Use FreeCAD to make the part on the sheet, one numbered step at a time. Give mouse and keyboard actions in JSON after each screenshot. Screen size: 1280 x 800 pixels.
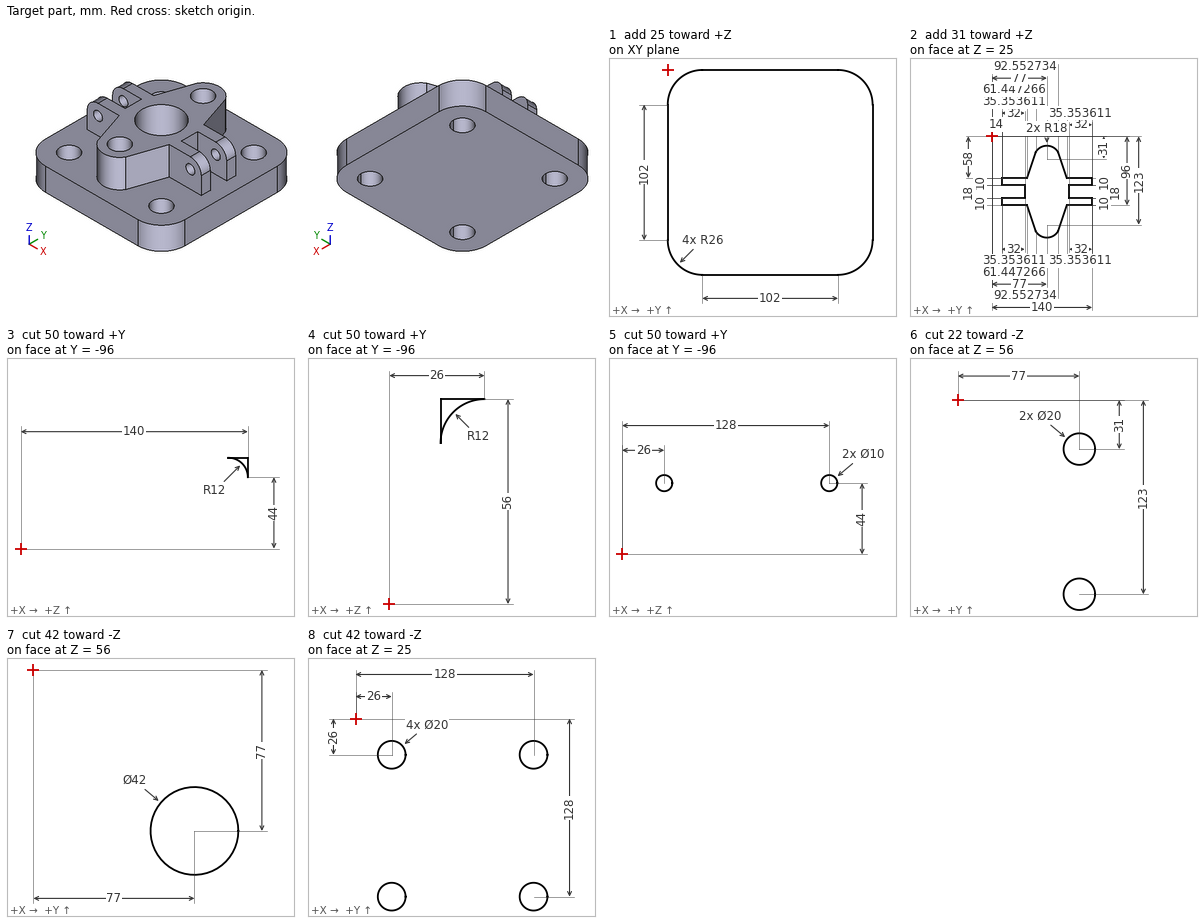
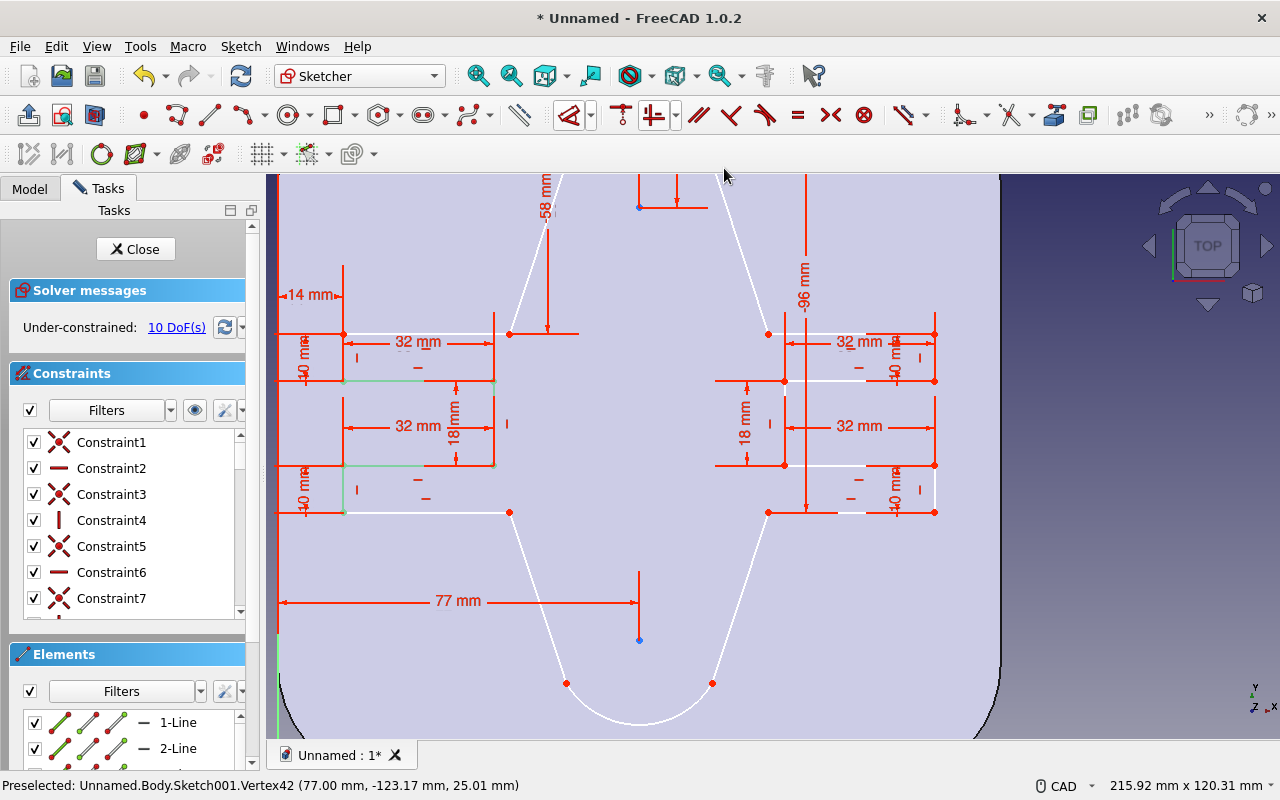
{"action": "left_click", "coordinate": [935, 513]}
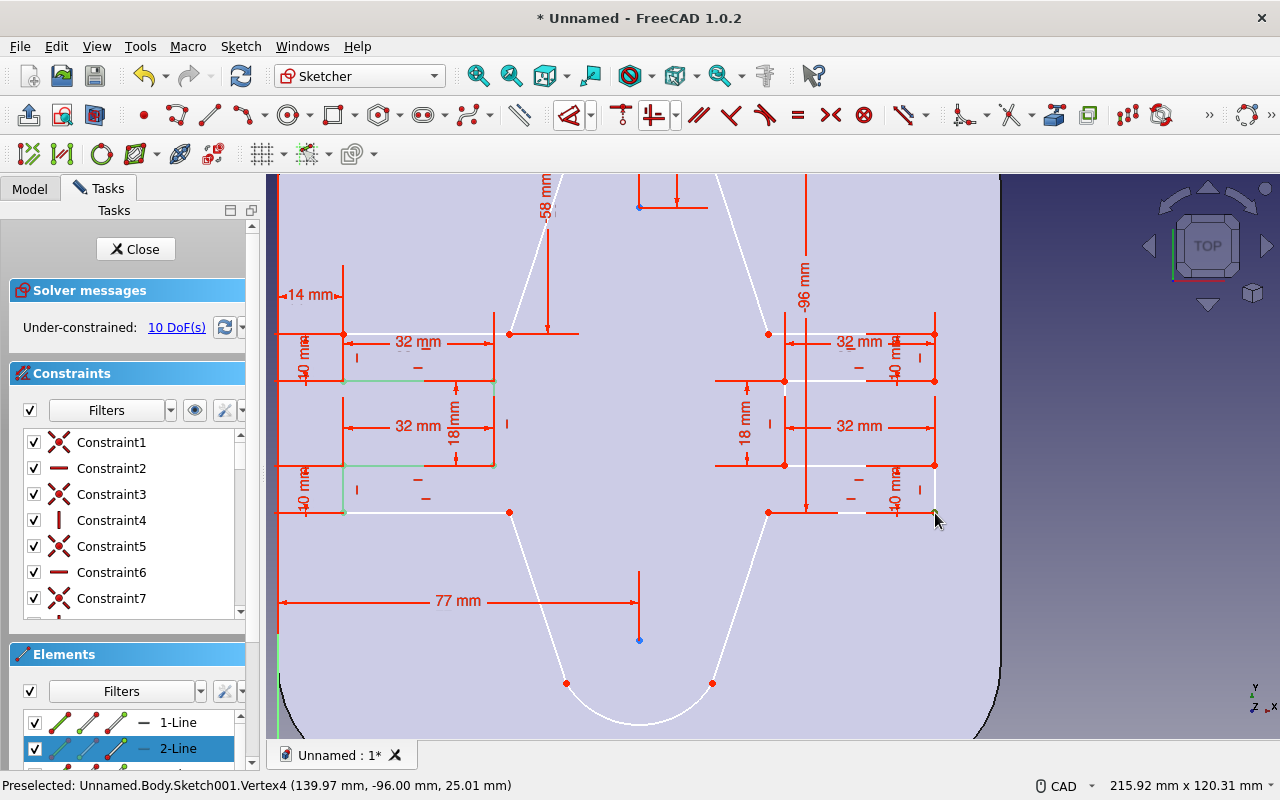
{"action": "key", "text": "l"}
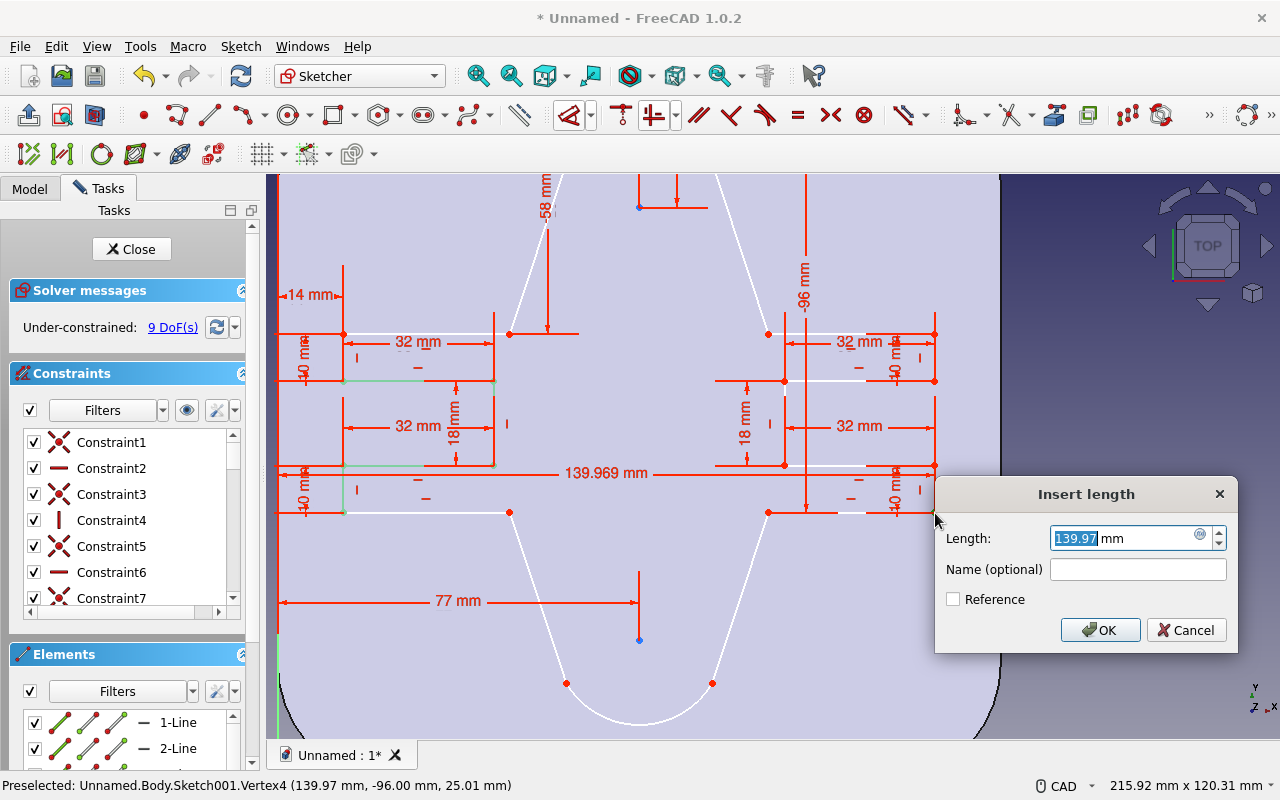
{"action": "type", "text": "140"}
{"action": "key", "text": "Return"}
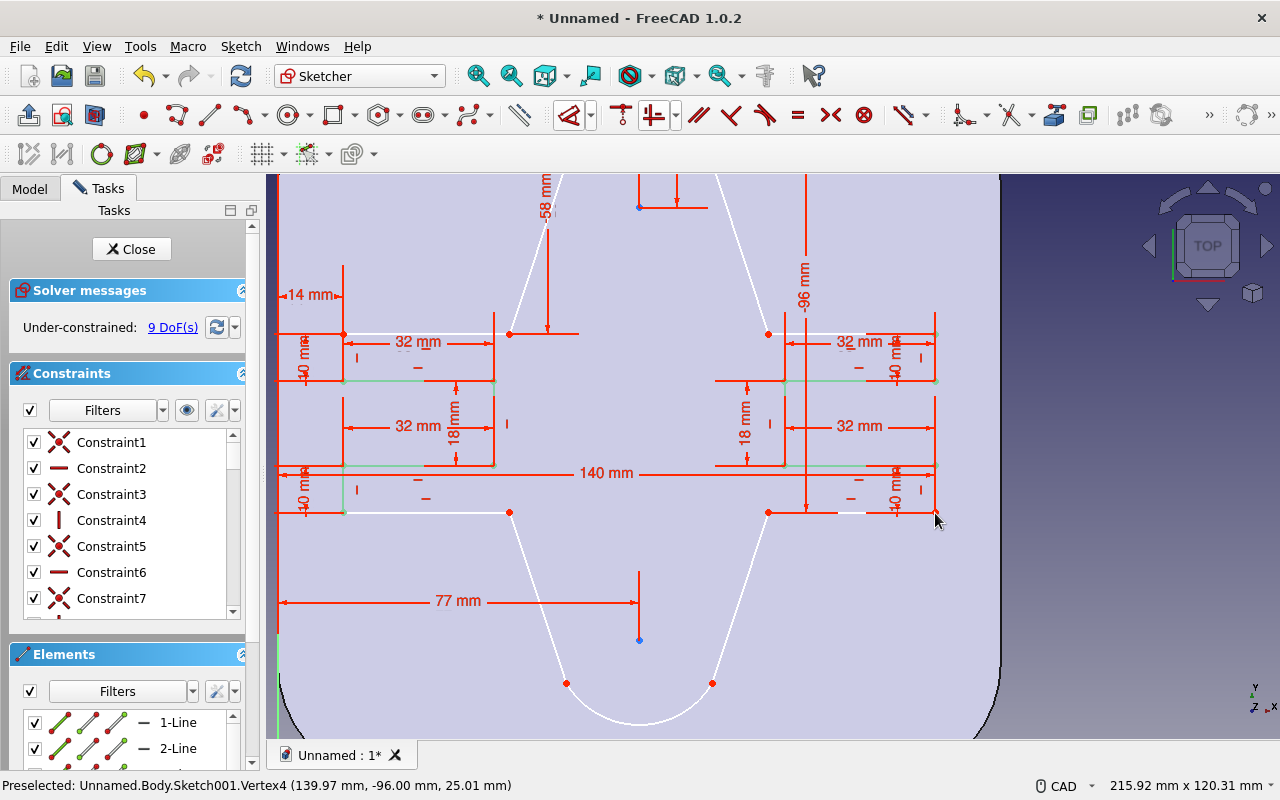
{"action": "left_click", "coordinate": [639, 640]}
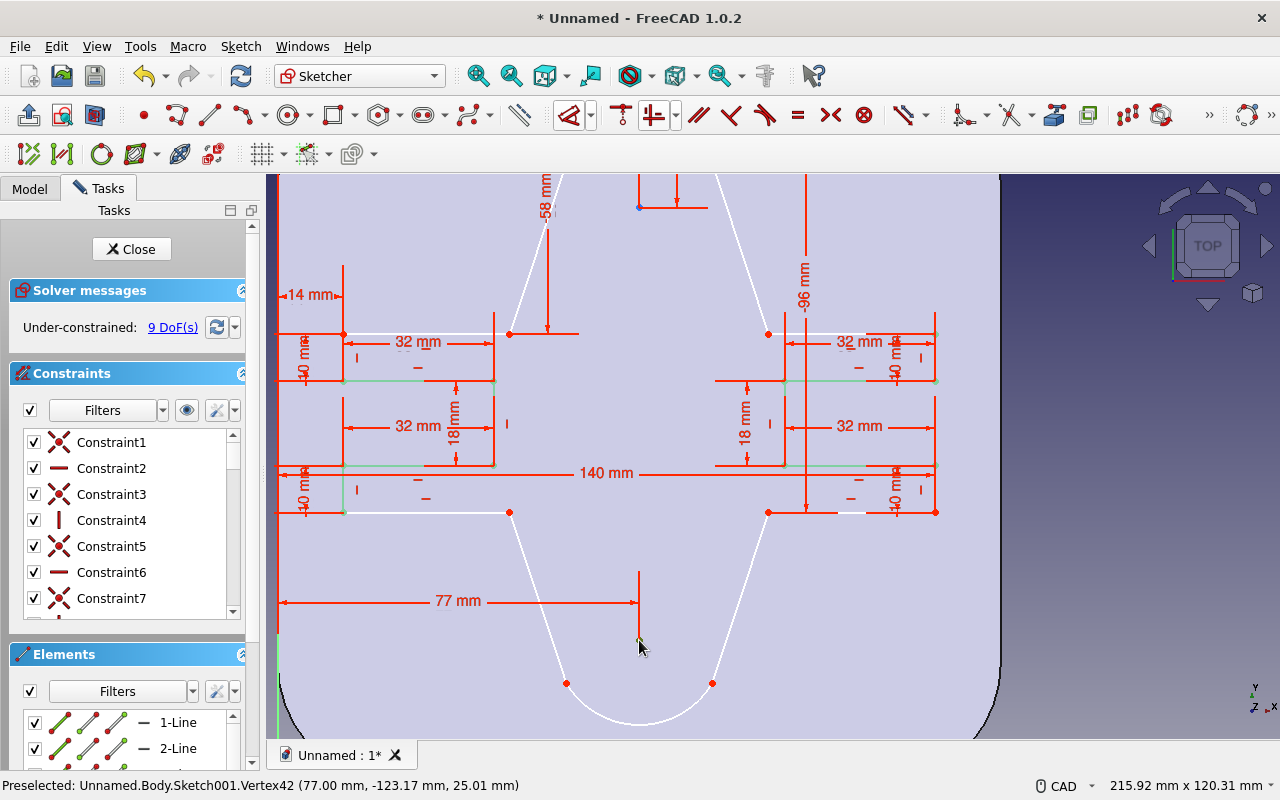
{"action": "key", "text": "i"}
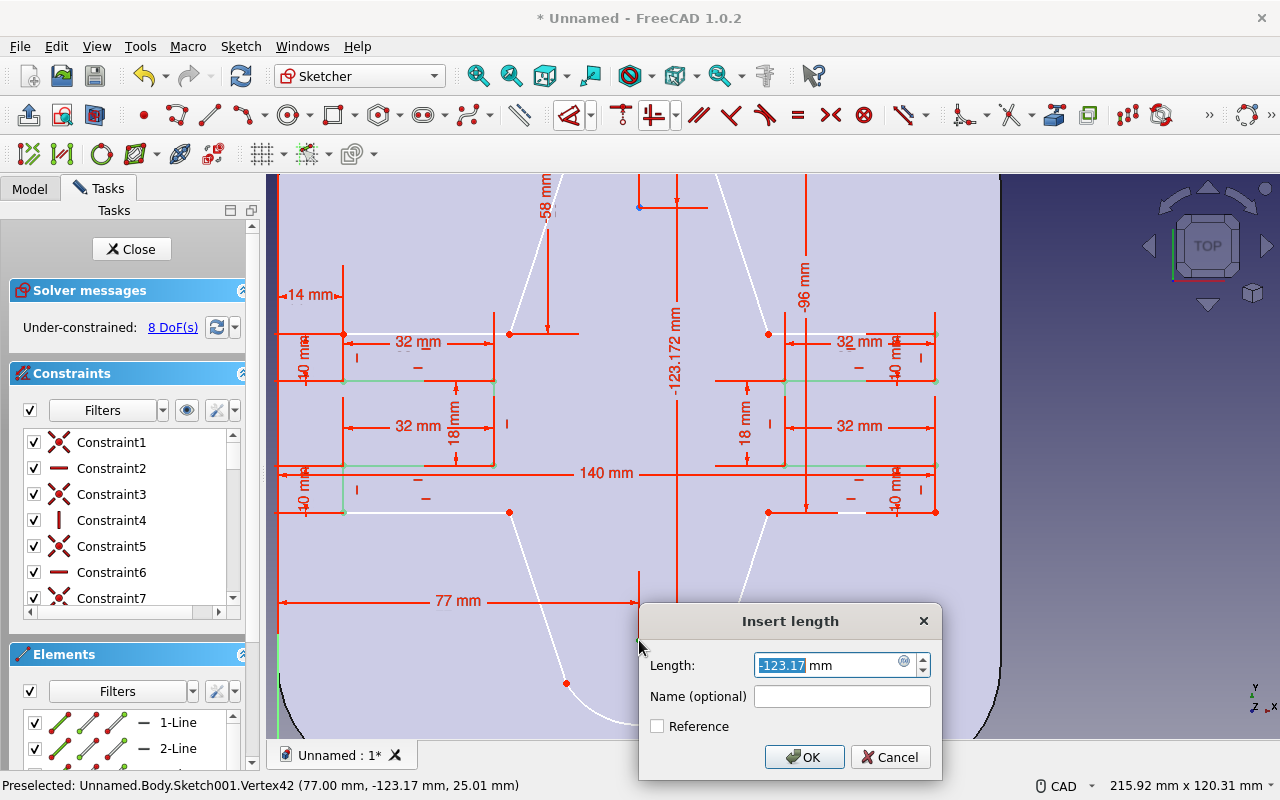
{"action": "type", "text": "-123"}
{"action": "key", "text": "Return"}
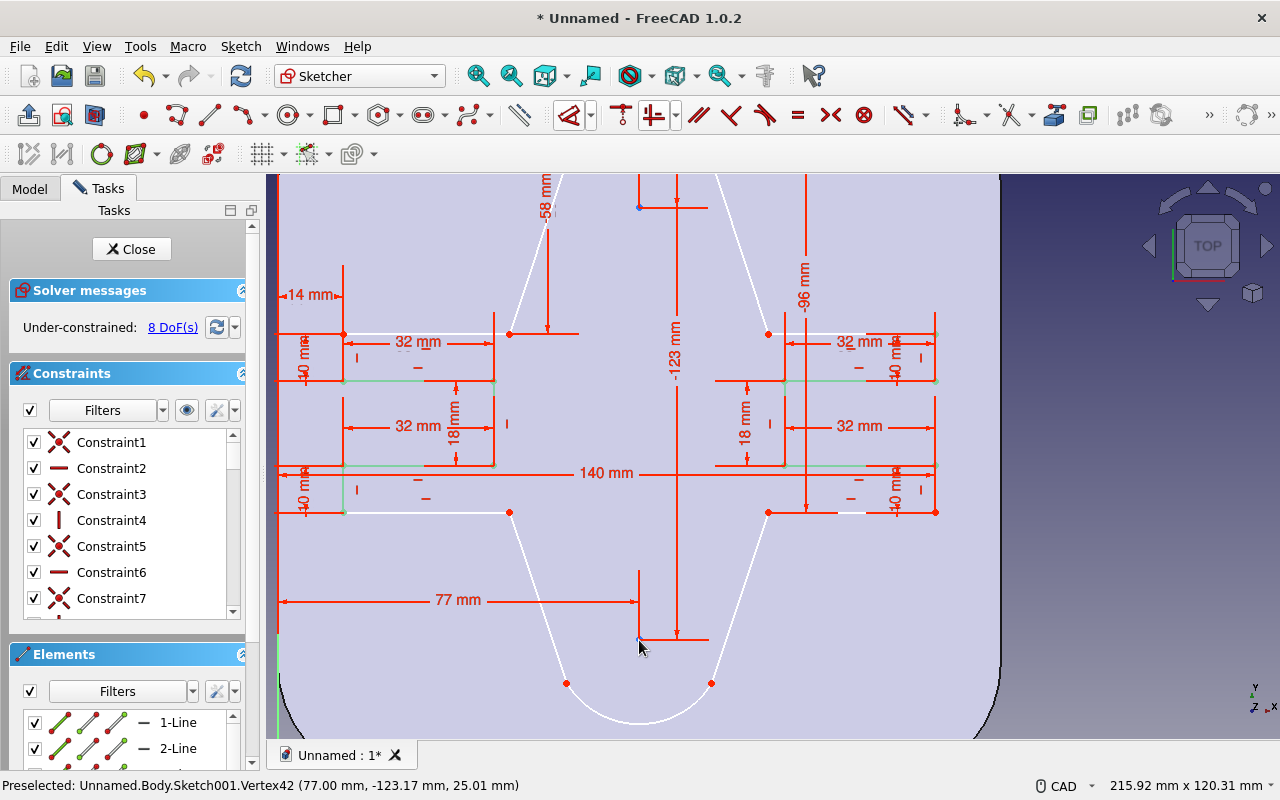
{"action": "left_click", "coordinate": [819, 513]}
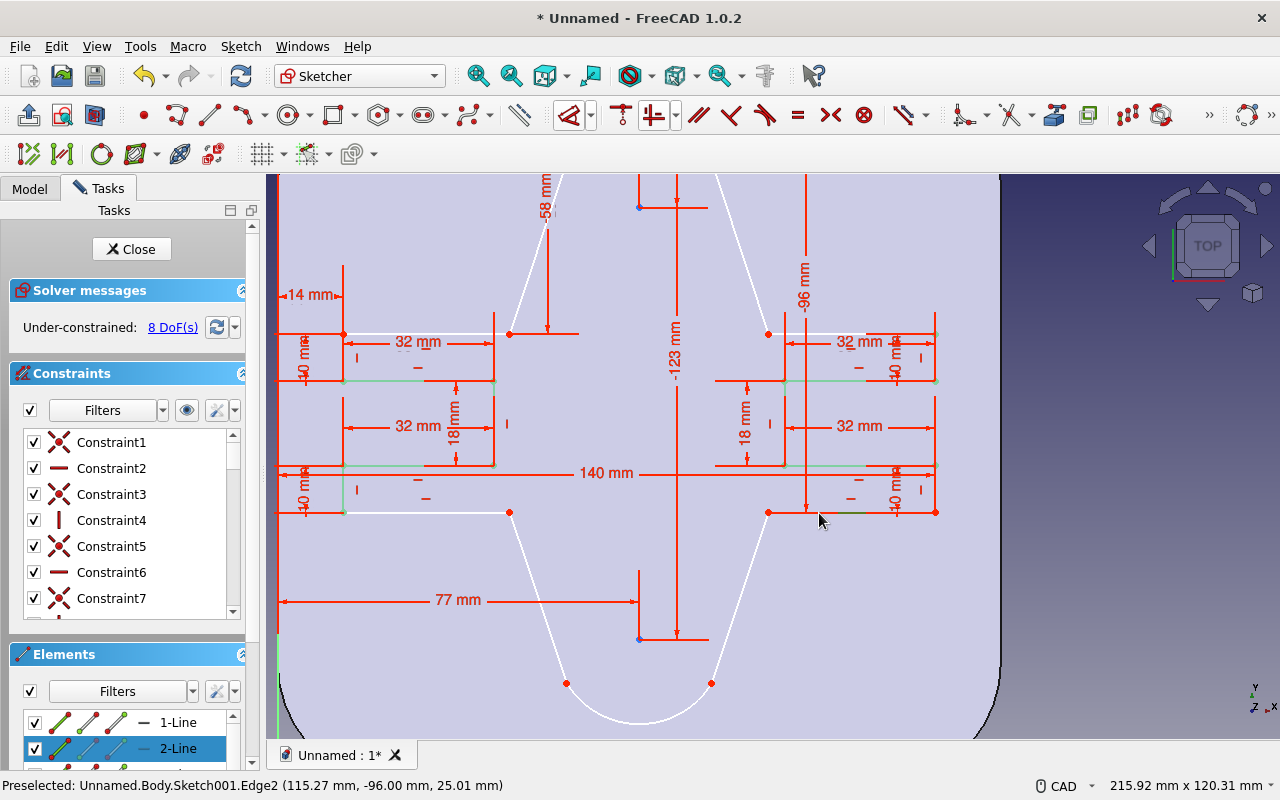
{"action": "left_click", "coordinate": [590, 116]}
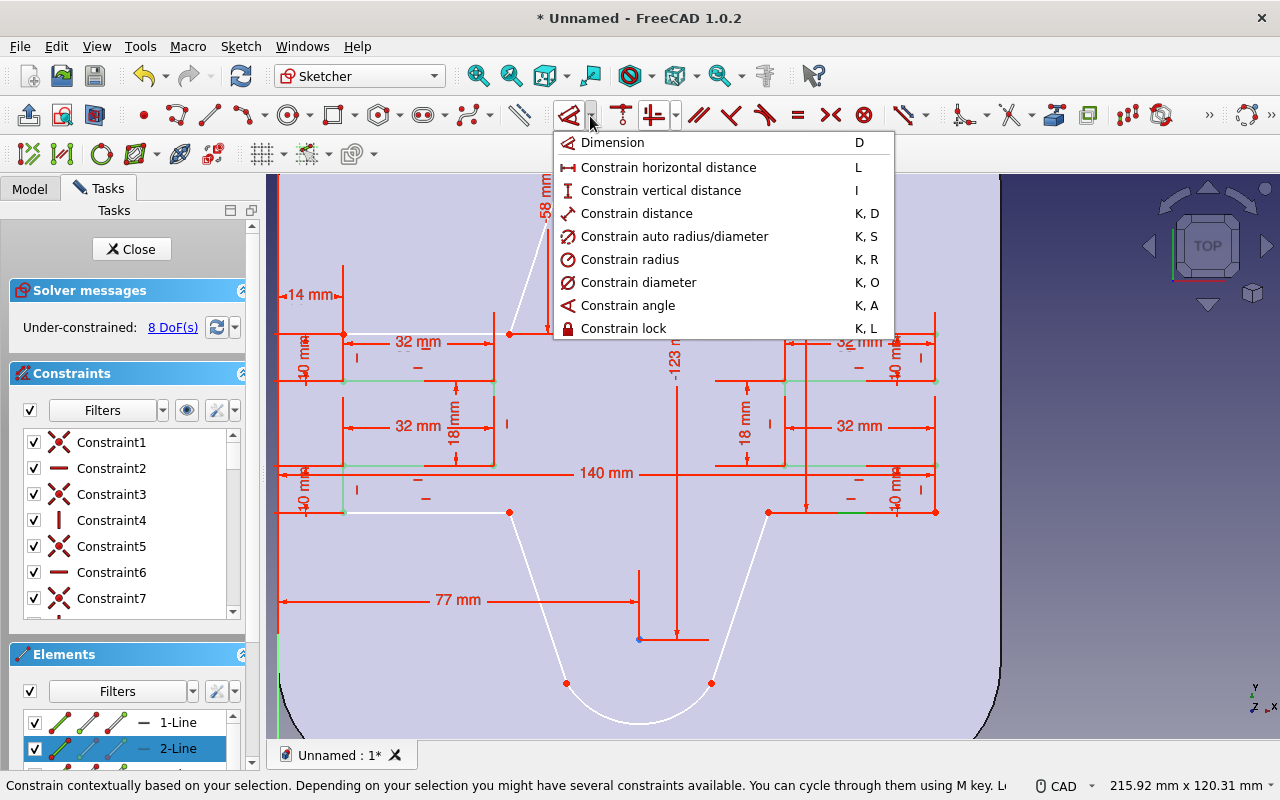
{"action": "left_click", "coordinate": [724, 168]}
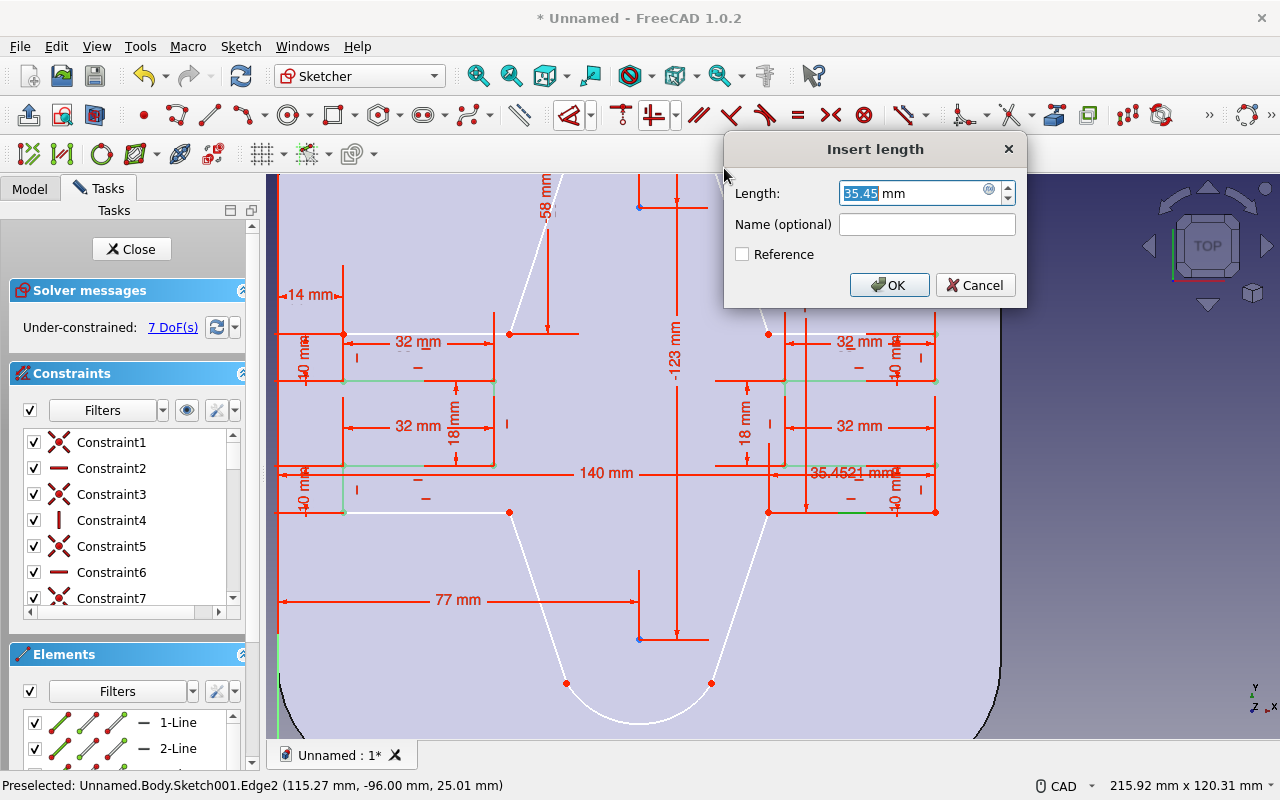
{"action": "type", "text": "35.353611"}
{"action": "key", "text": "Return"}